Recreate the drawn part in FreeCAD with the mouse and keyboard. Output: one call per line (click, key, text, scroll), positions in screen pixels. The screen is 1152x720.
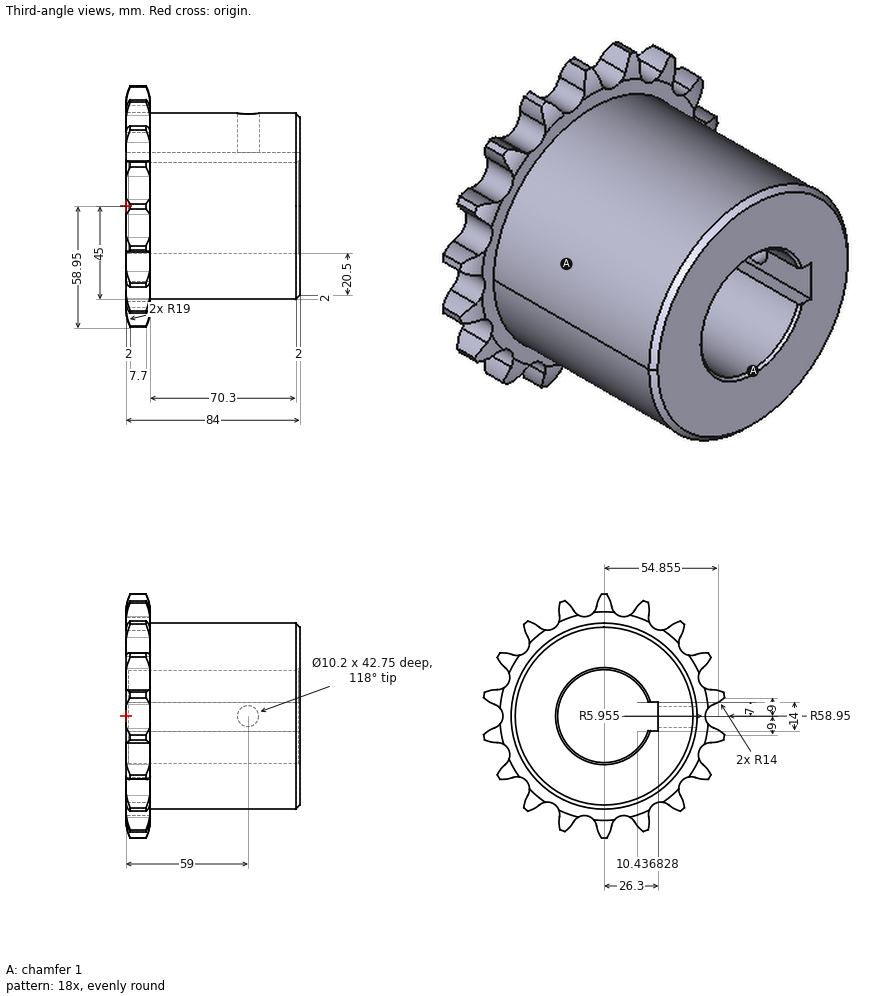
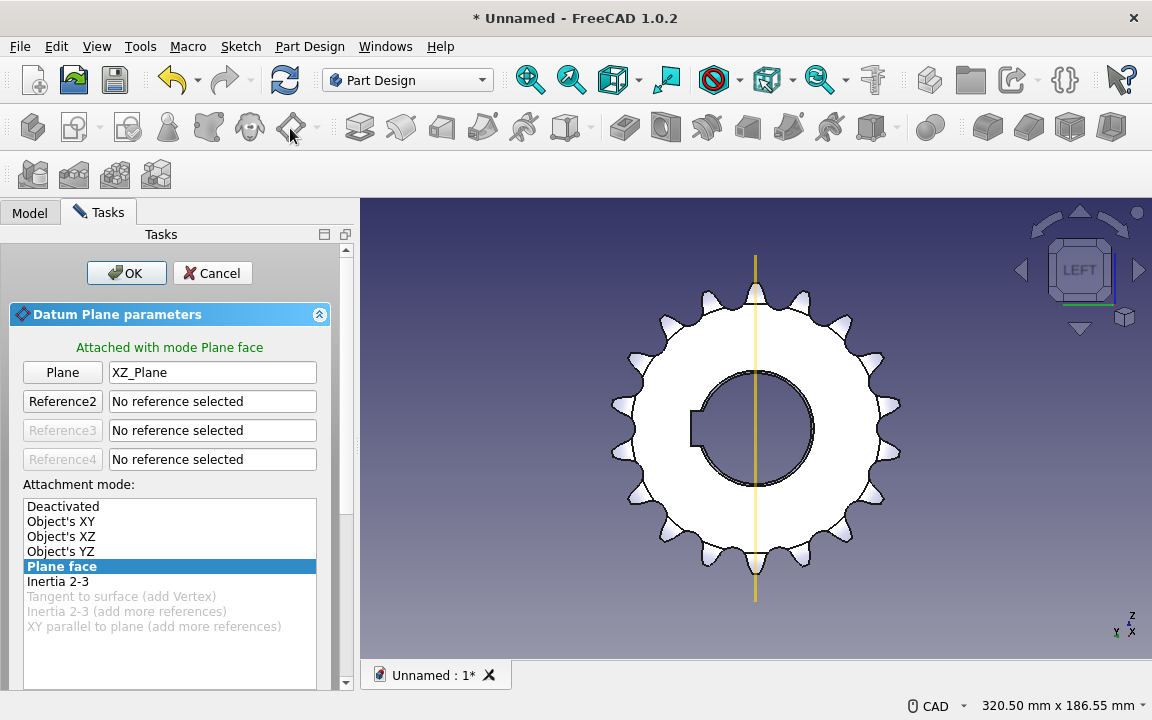
scroll(346, 467, down, 4)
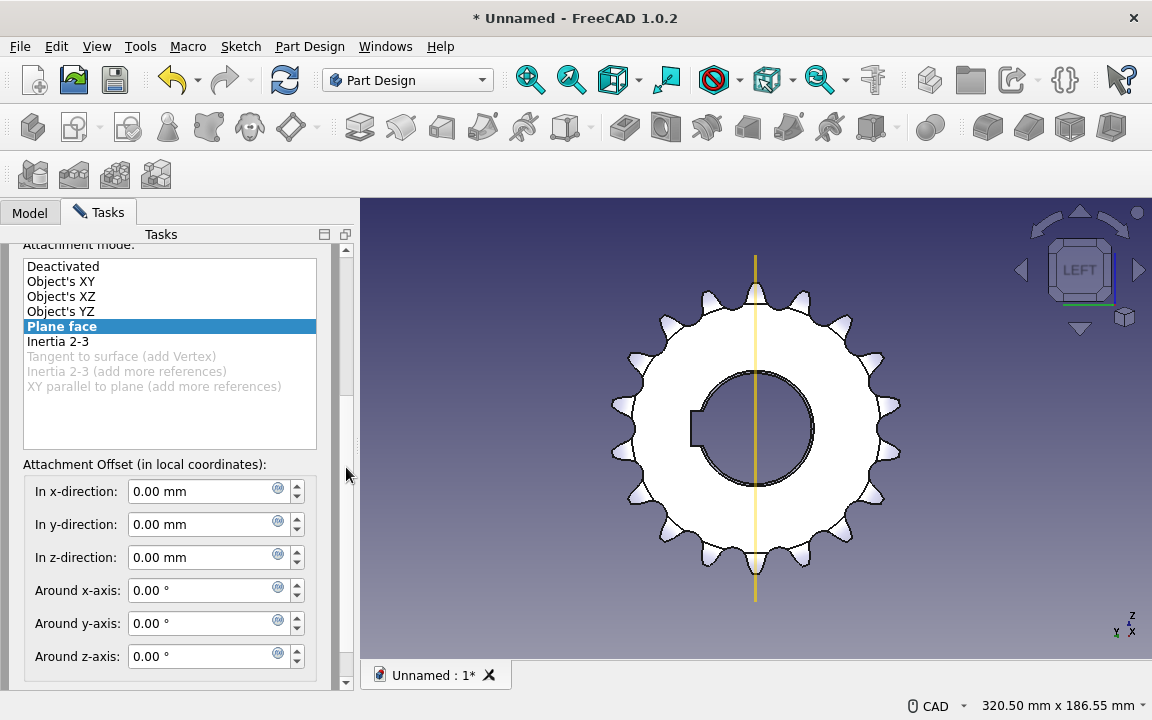
triple_click(210, 558)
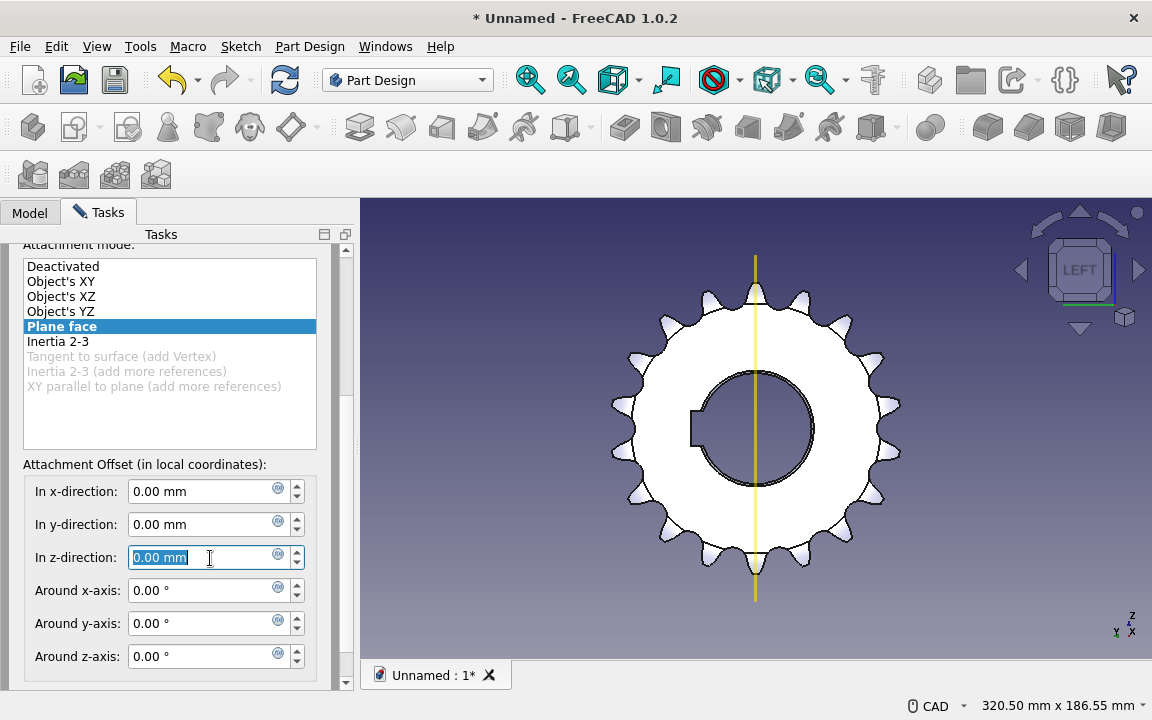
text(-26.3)
key(Tab)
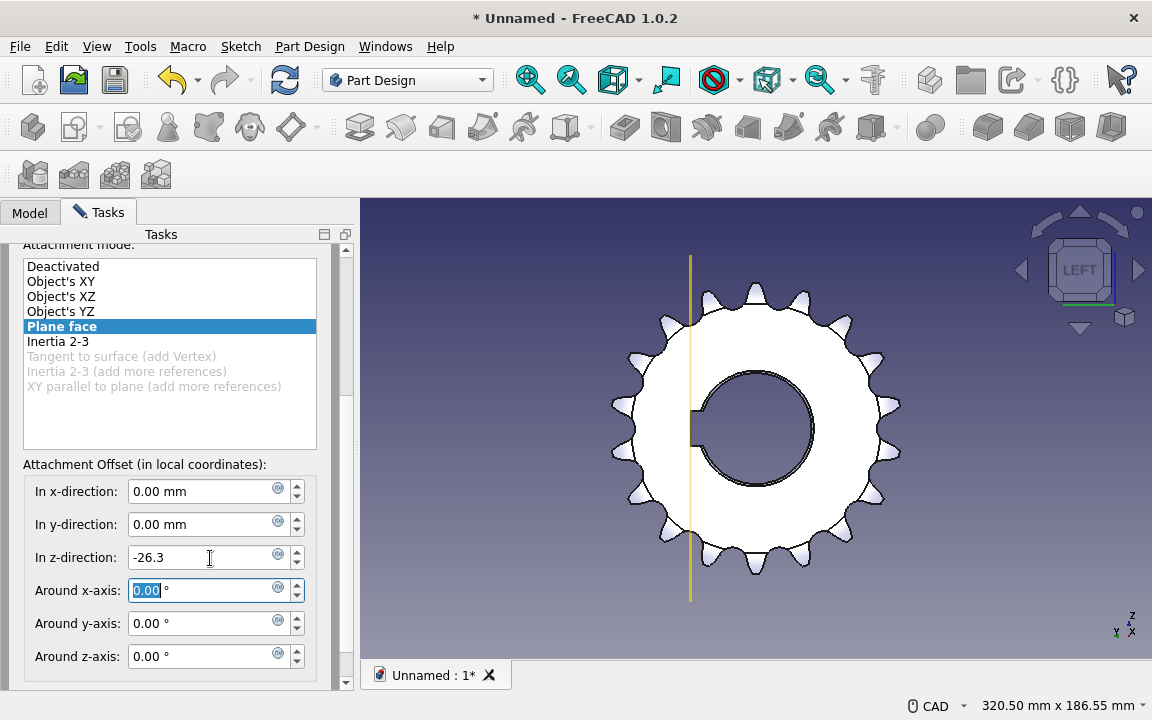
scroll(346, 467, up, 5)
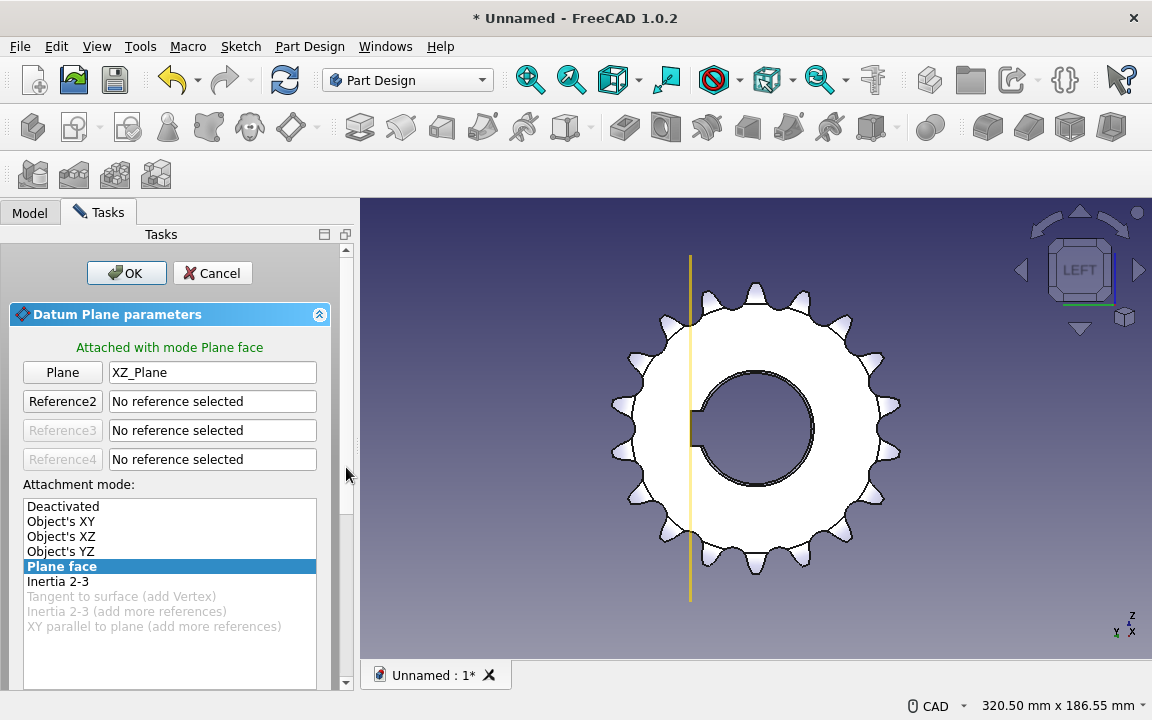
click(127, 273)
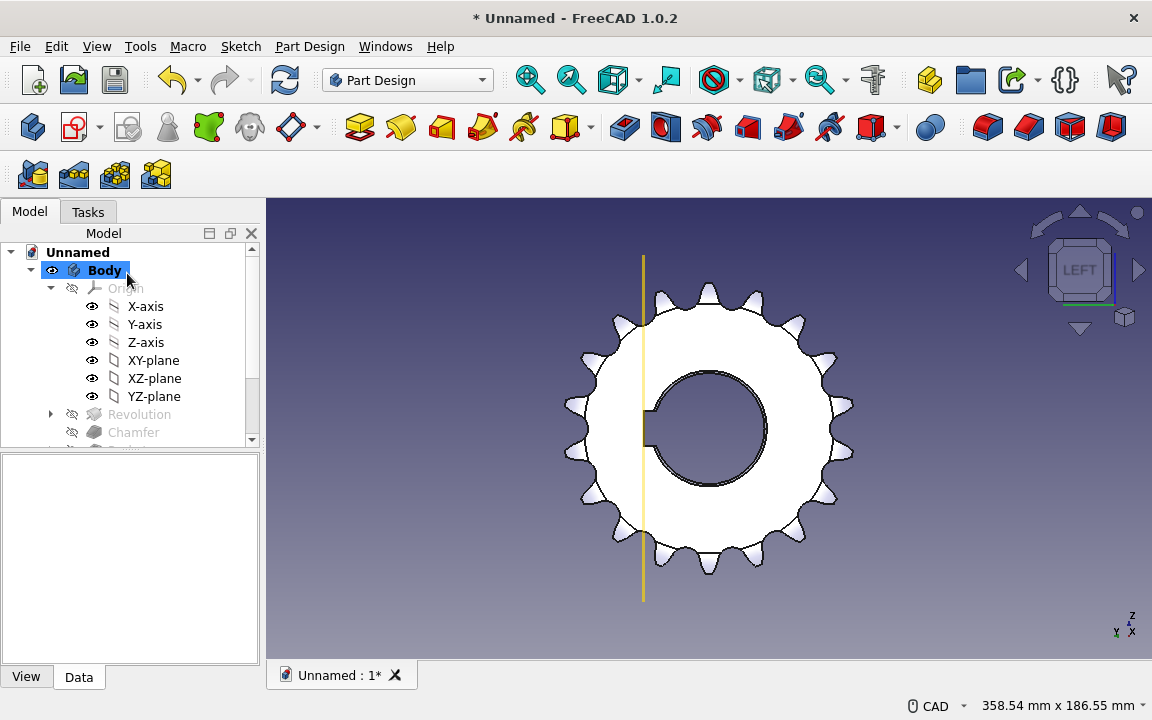
scroll(101, 338, down, 3)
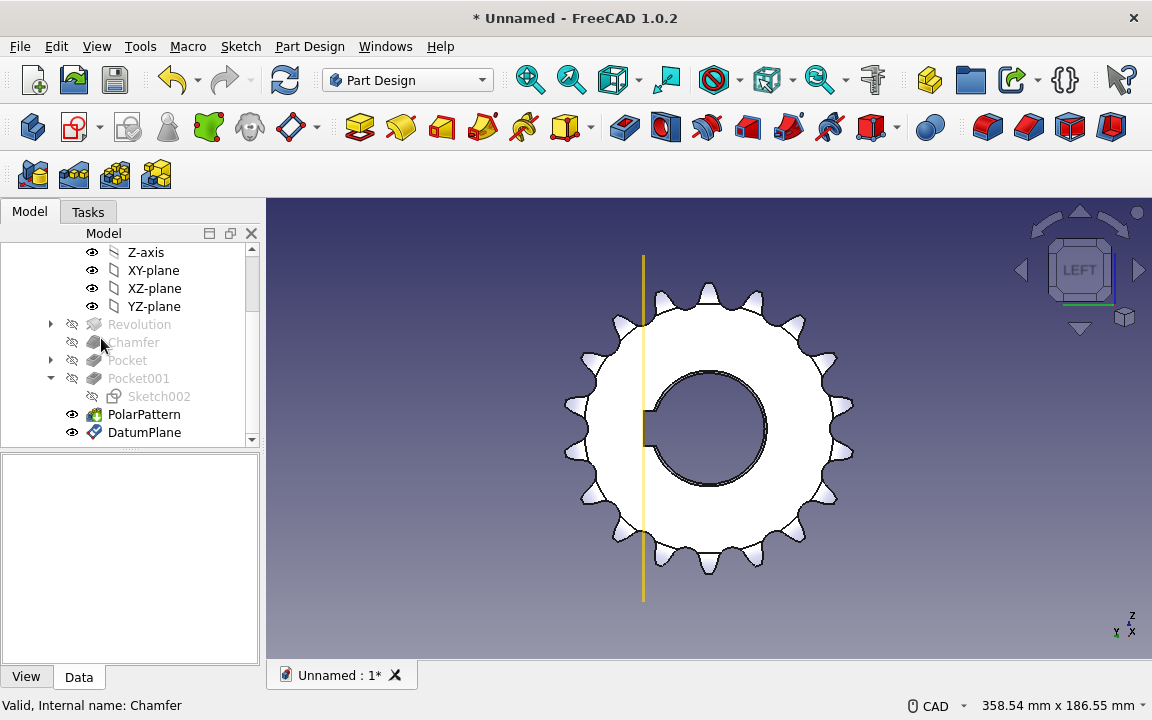
click(117, 432)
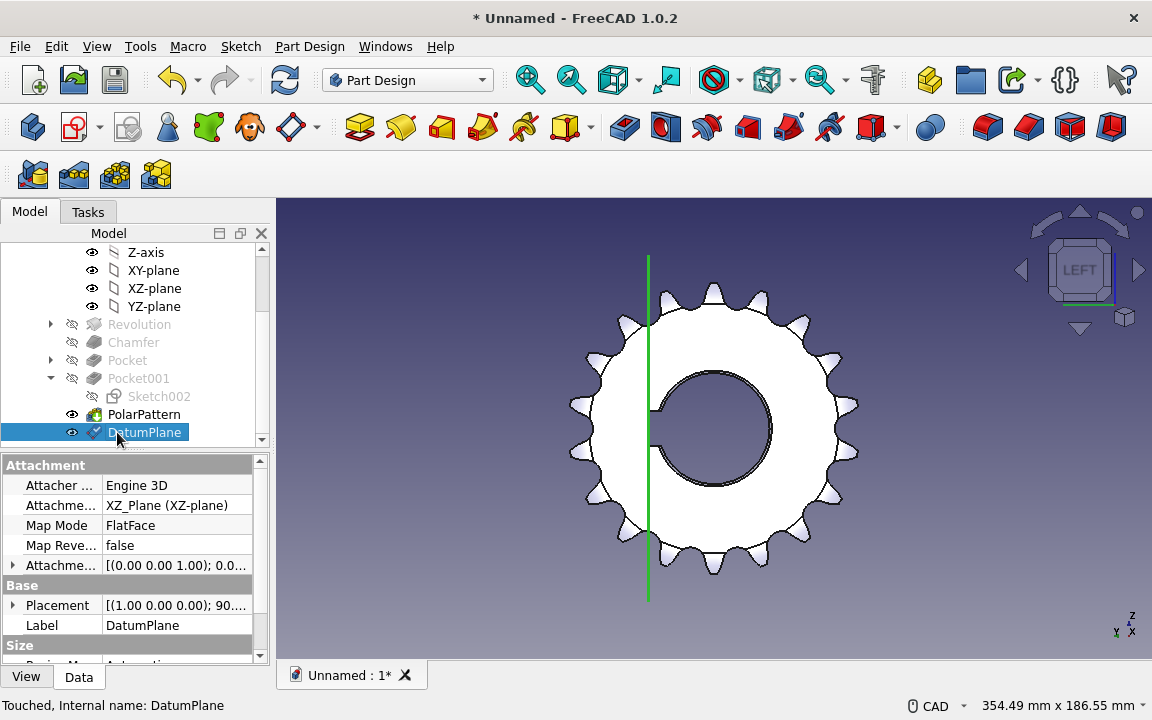
click(74, 128)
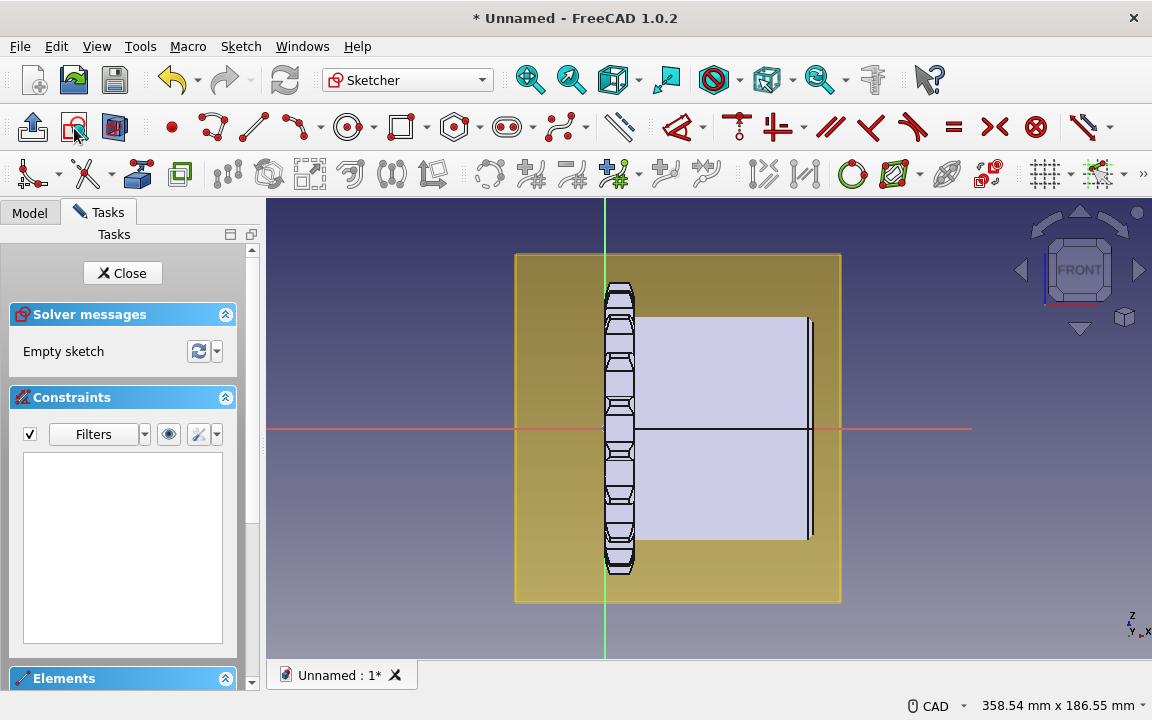
click(115, 128)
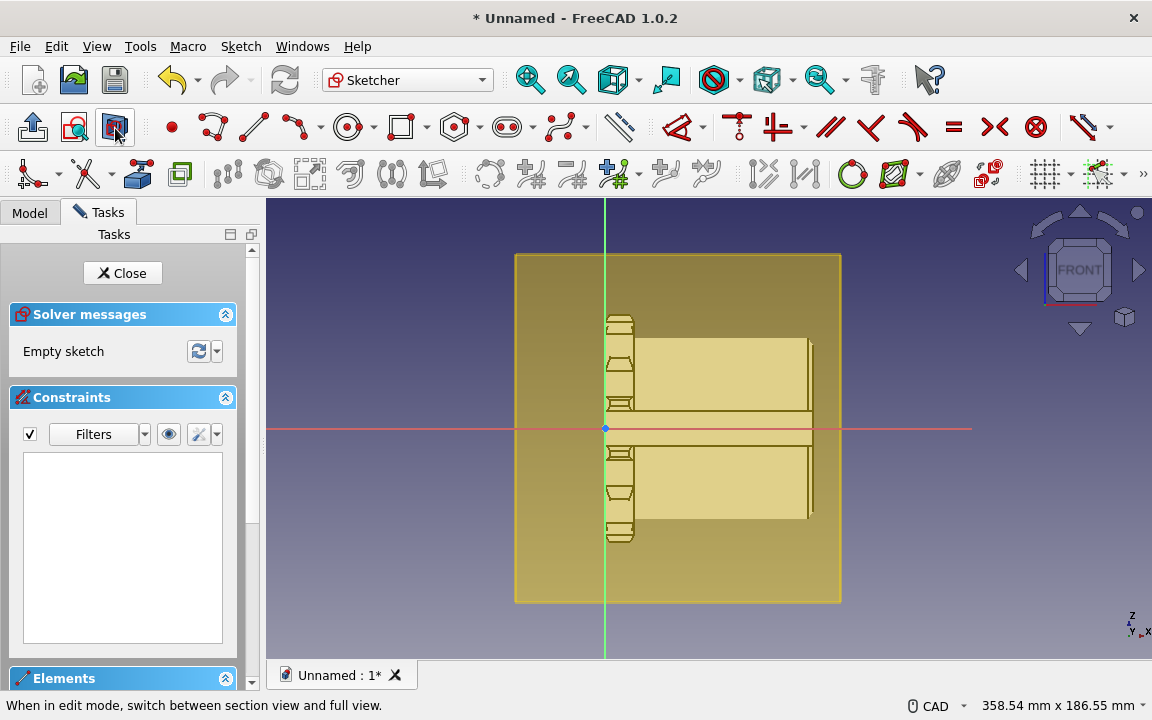
scroll(762, 429, up, 12)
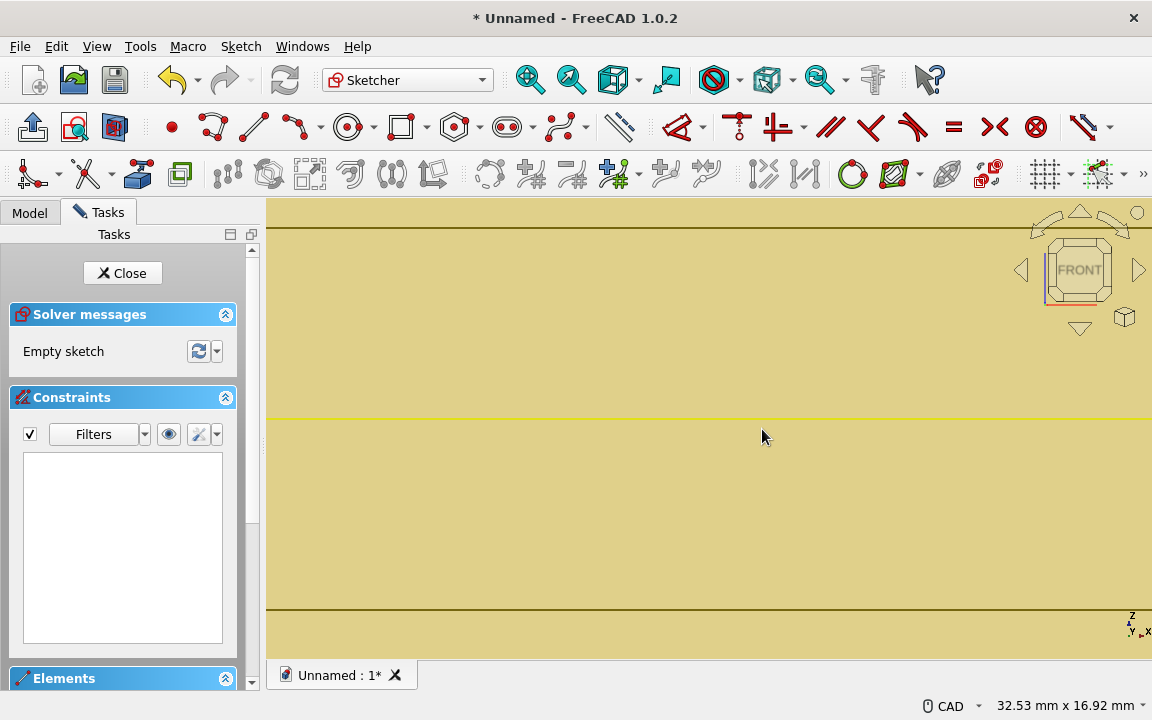
click(348, 128)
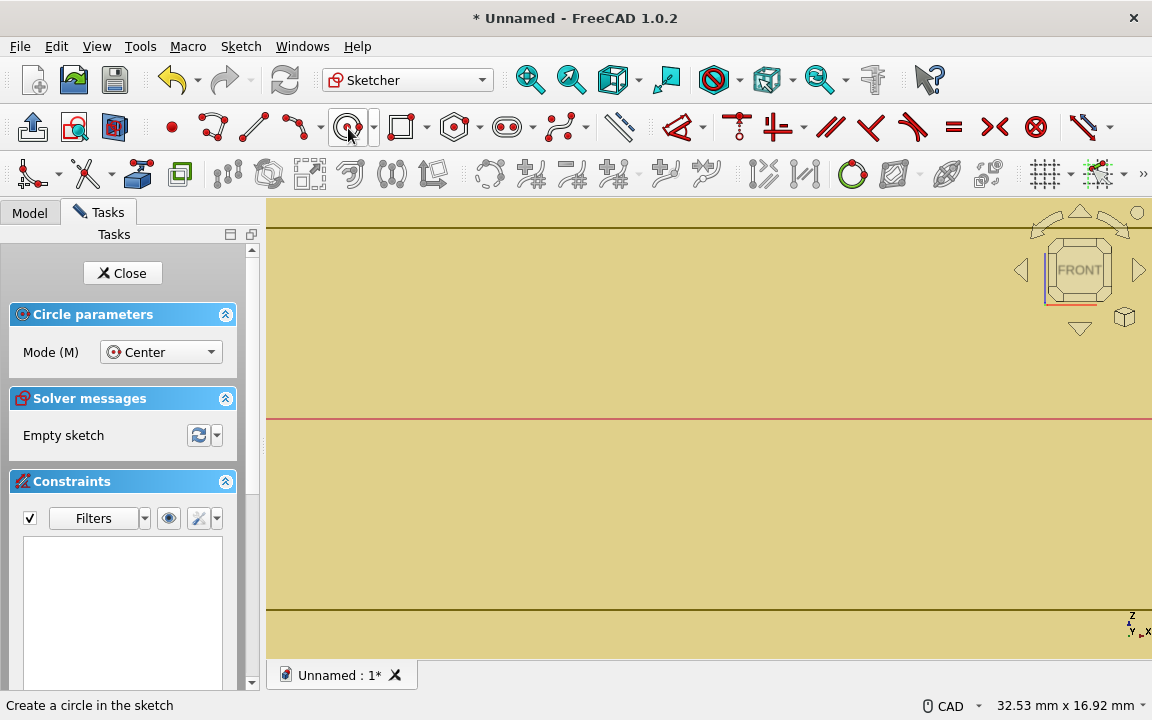
click(635, 419)
click(733, 321)
key(Escape)